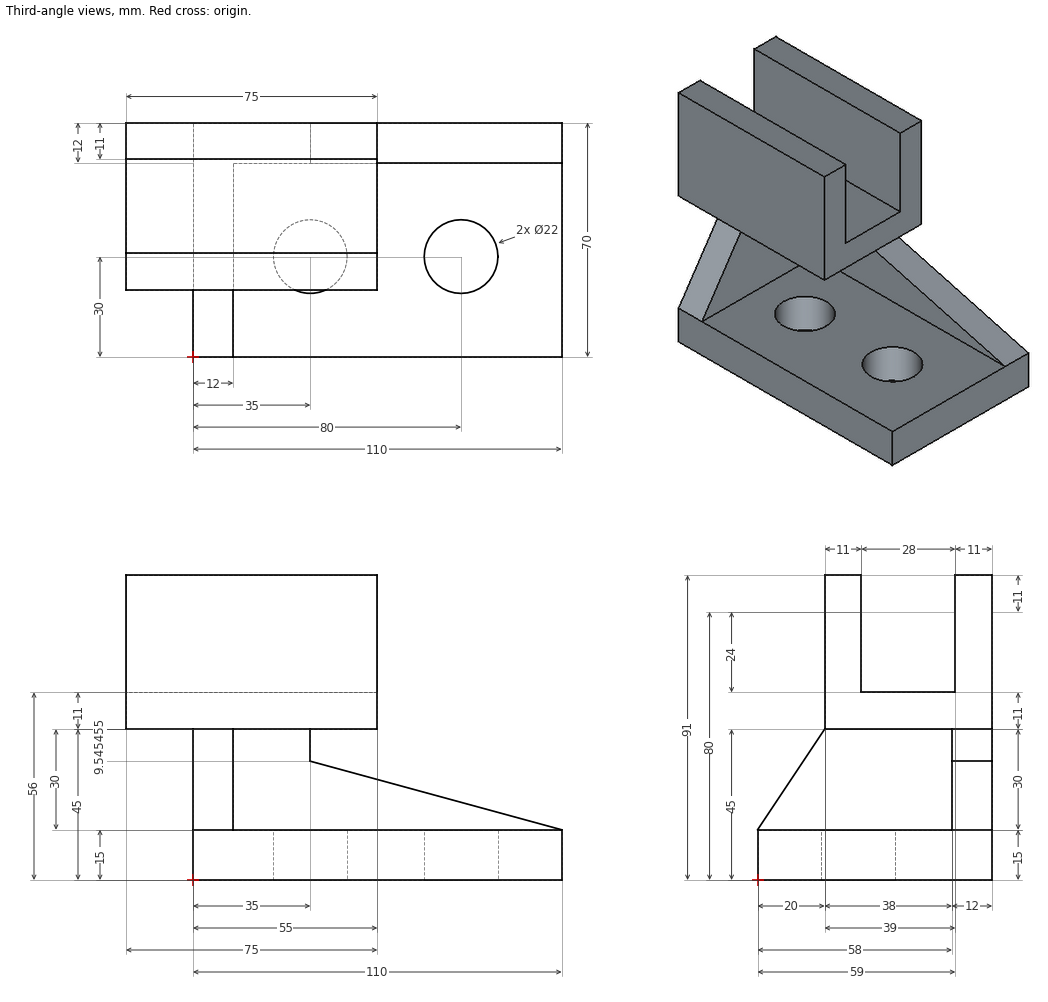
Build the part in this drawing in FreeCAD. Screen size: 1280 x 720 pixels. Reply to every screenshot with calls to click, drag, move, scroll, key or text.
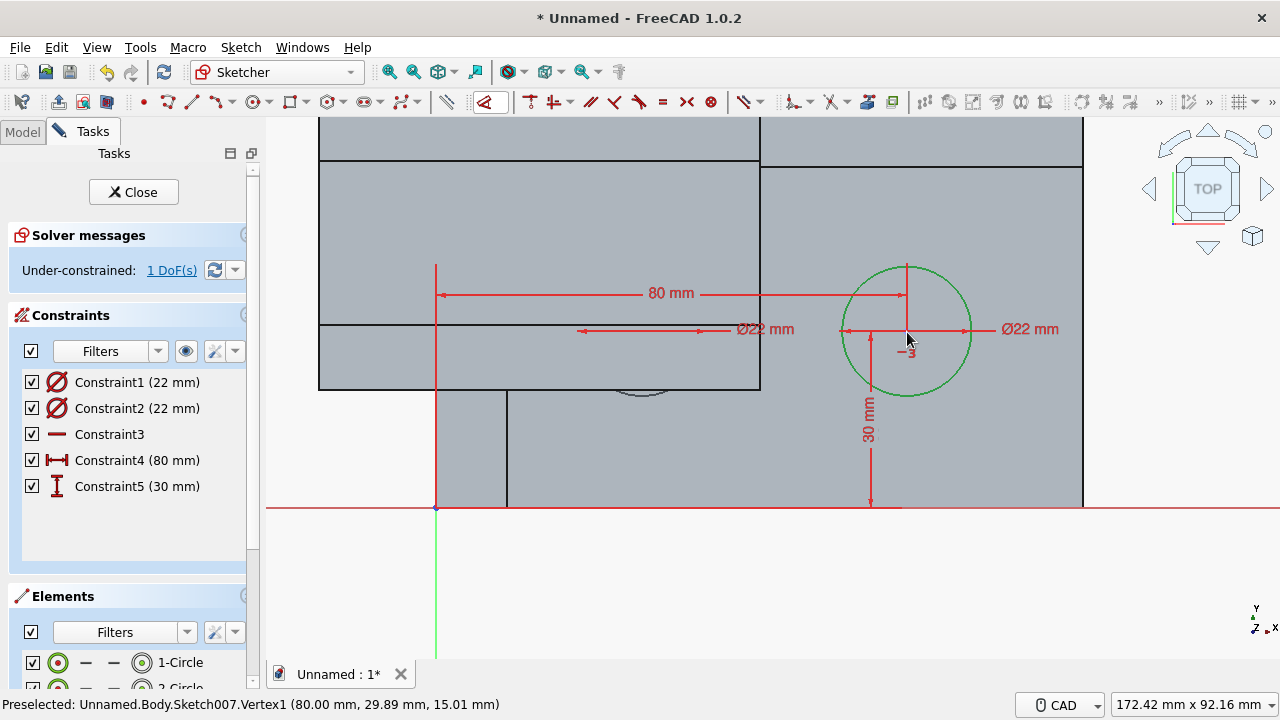
click(642, 331)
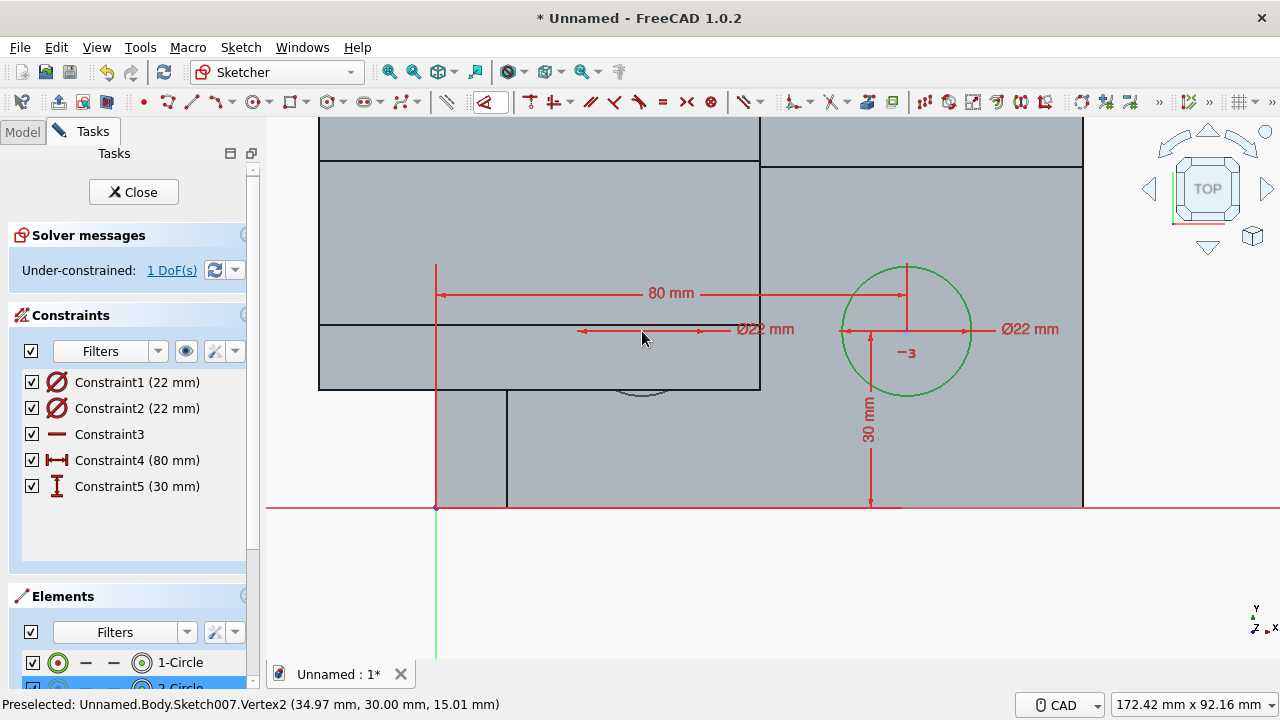
key(l)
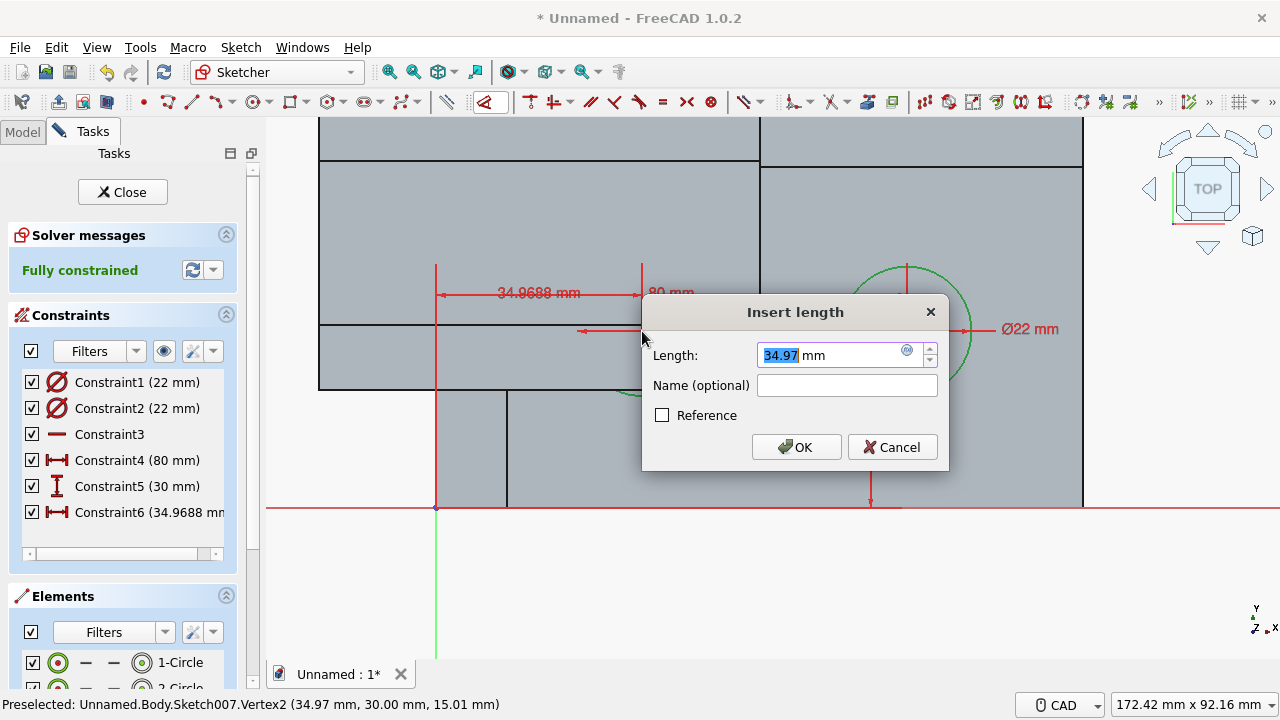
text(35)
key(Return)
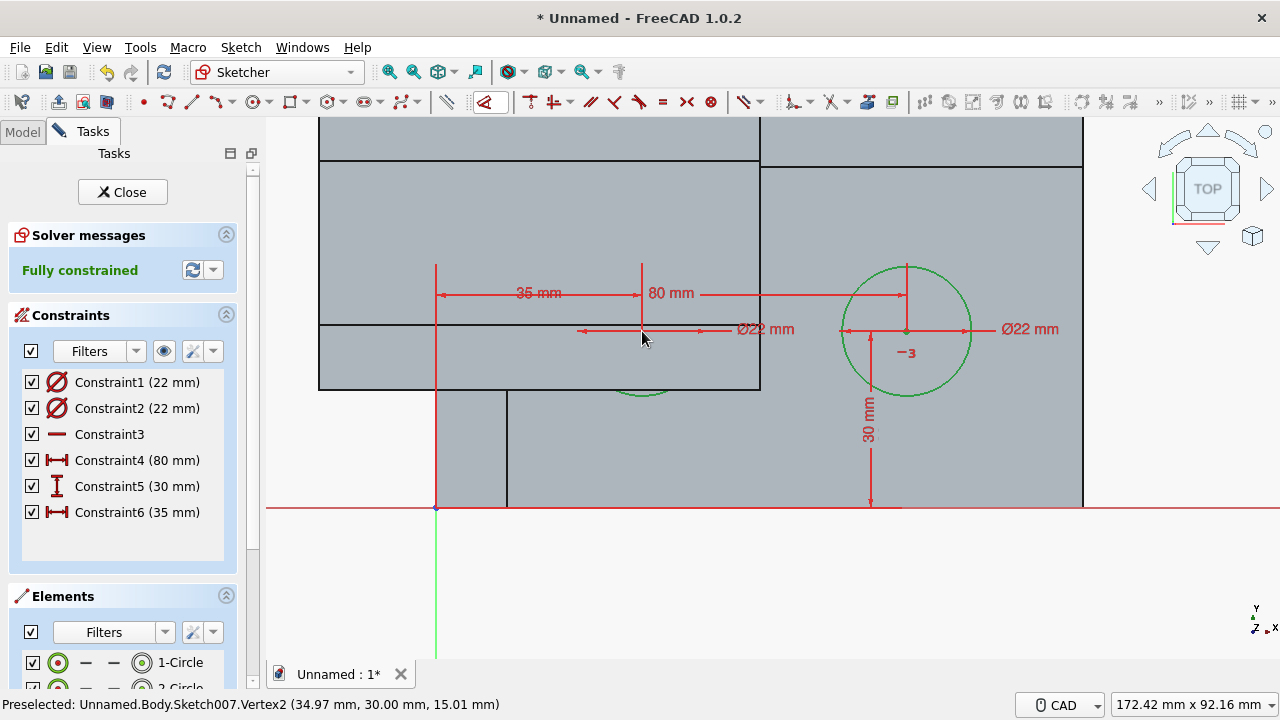
click(123, 192)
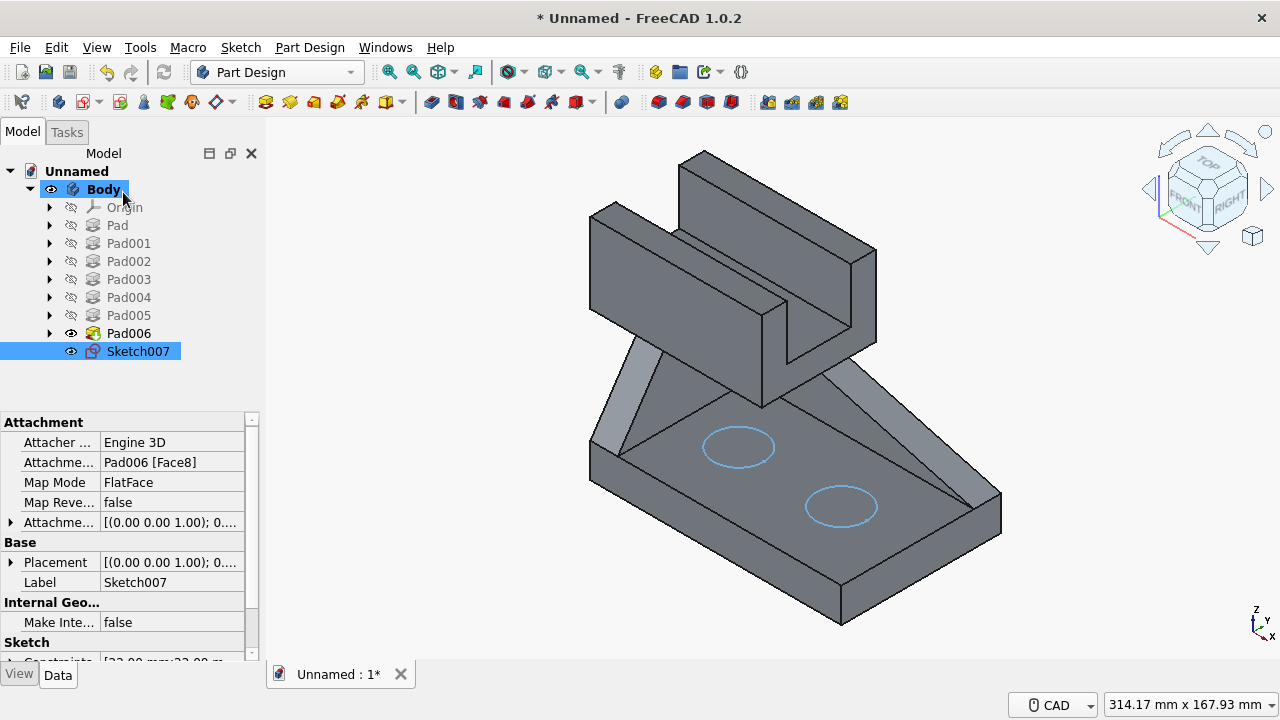
click(432, 102)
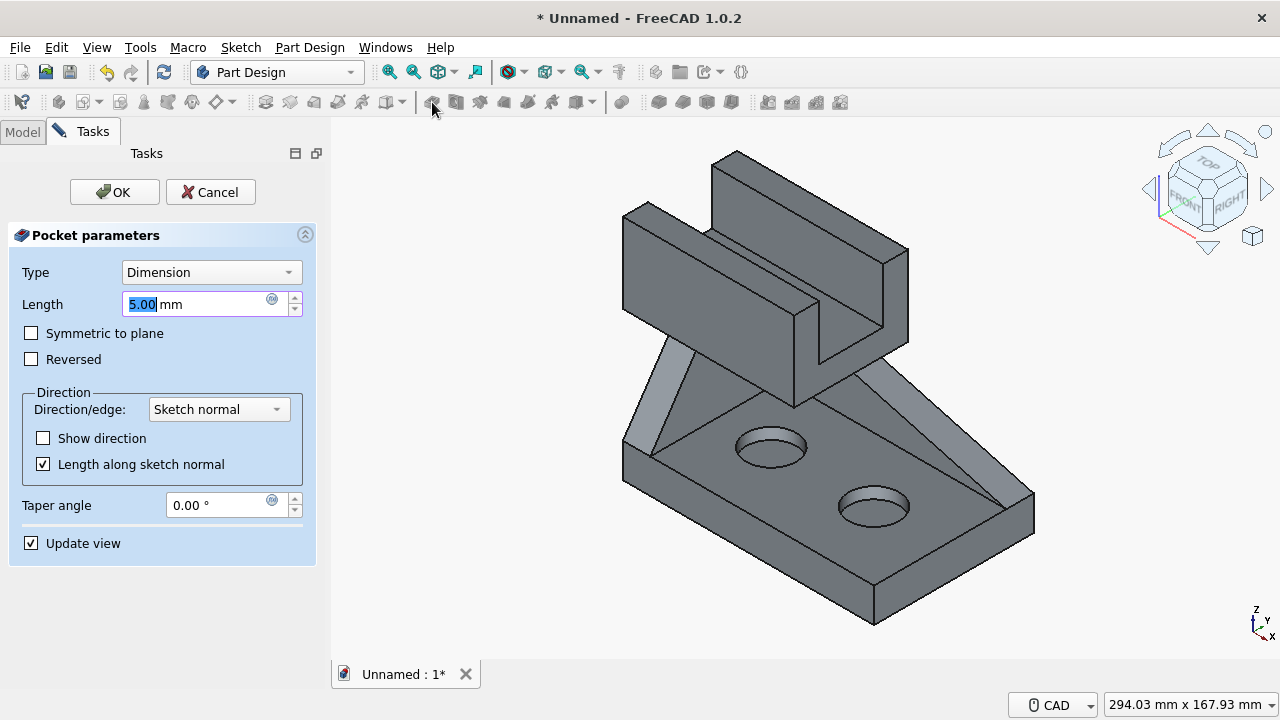
text(15)
key(Tab)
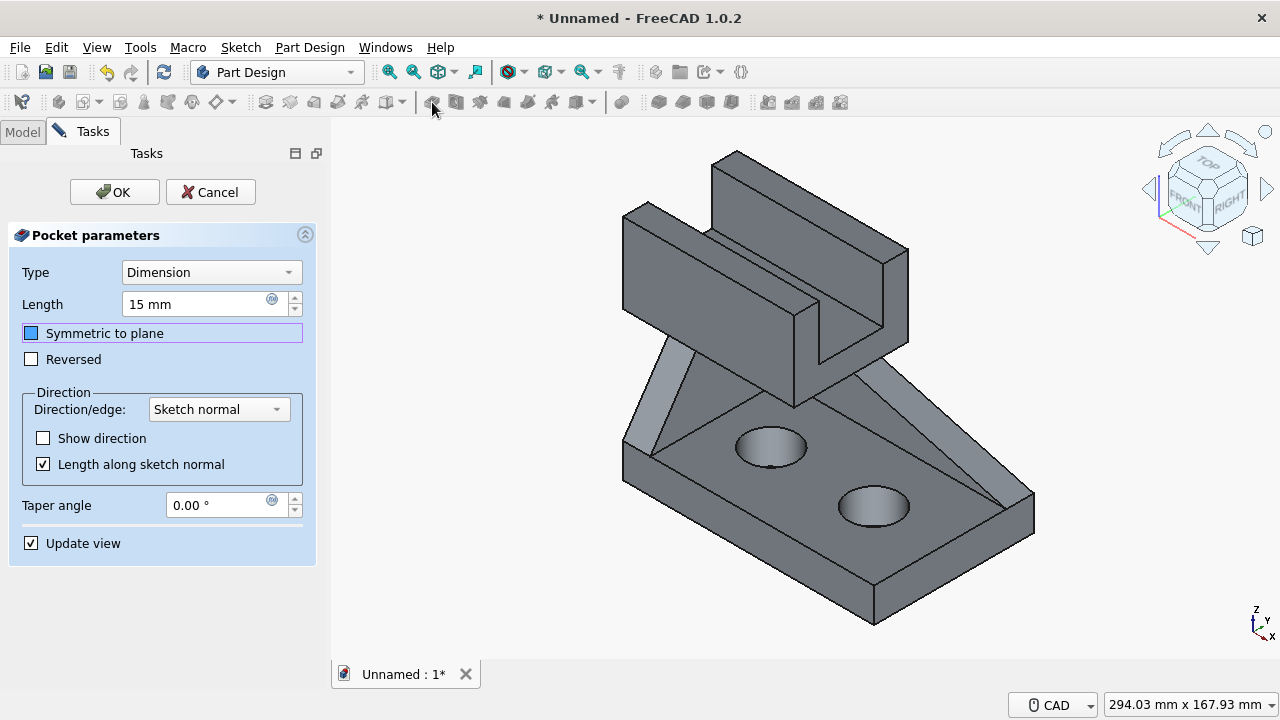
click(115, 192)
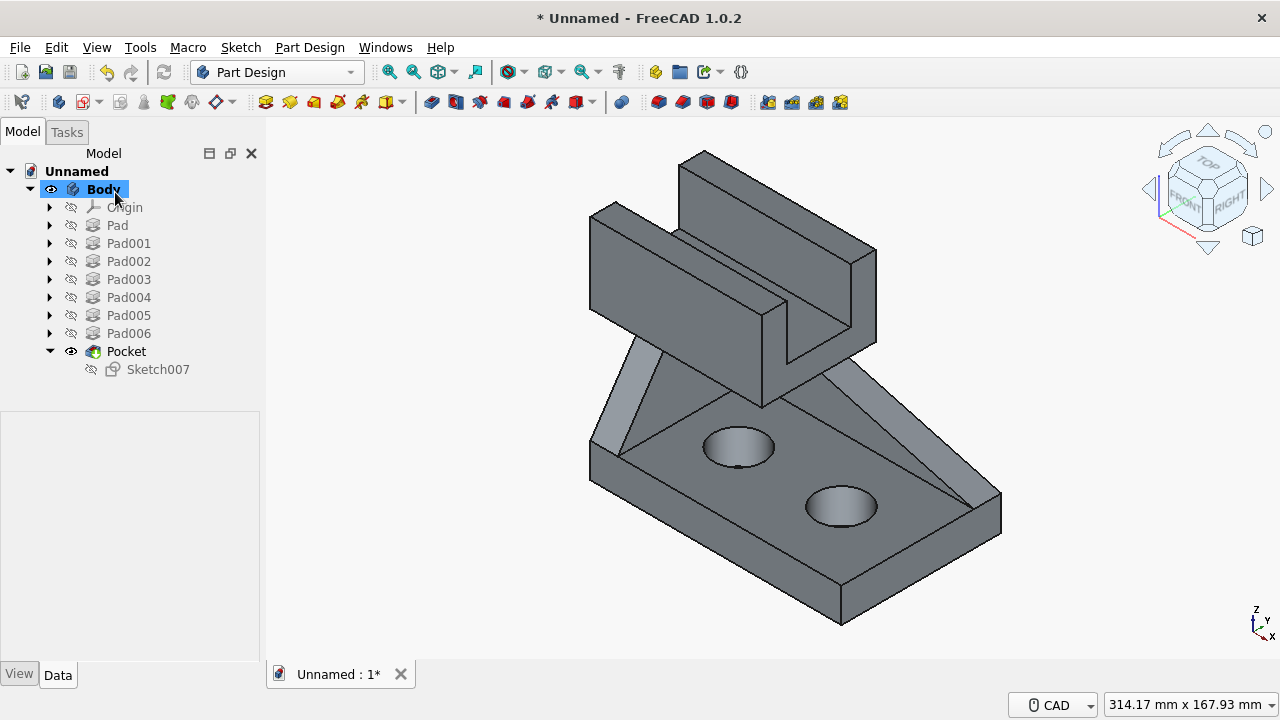
click(770, 330)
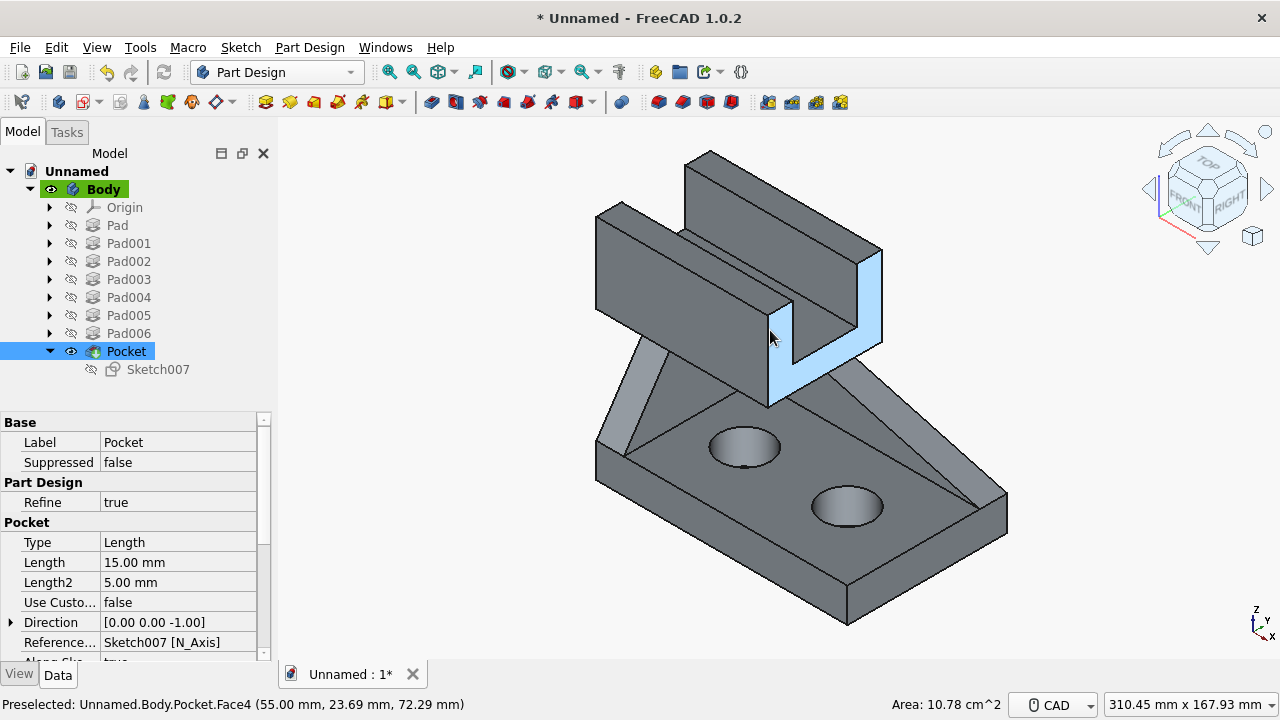
click(84, 102)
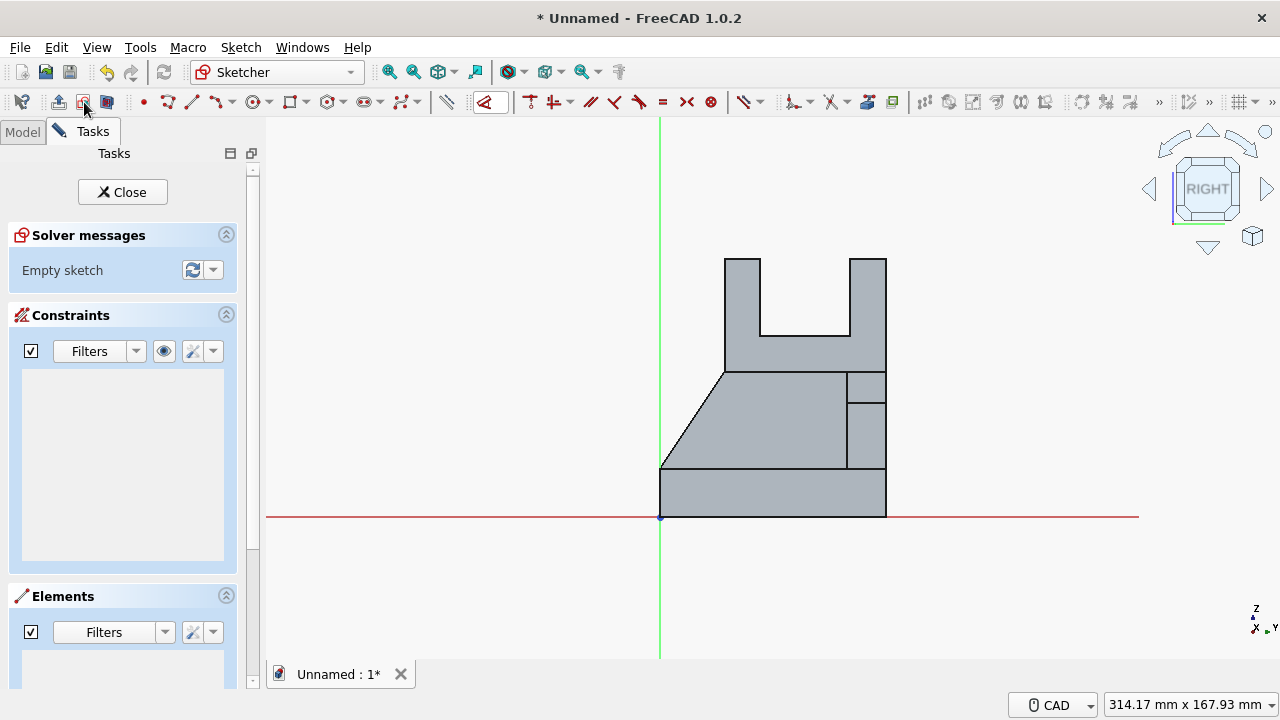
click(108, 102)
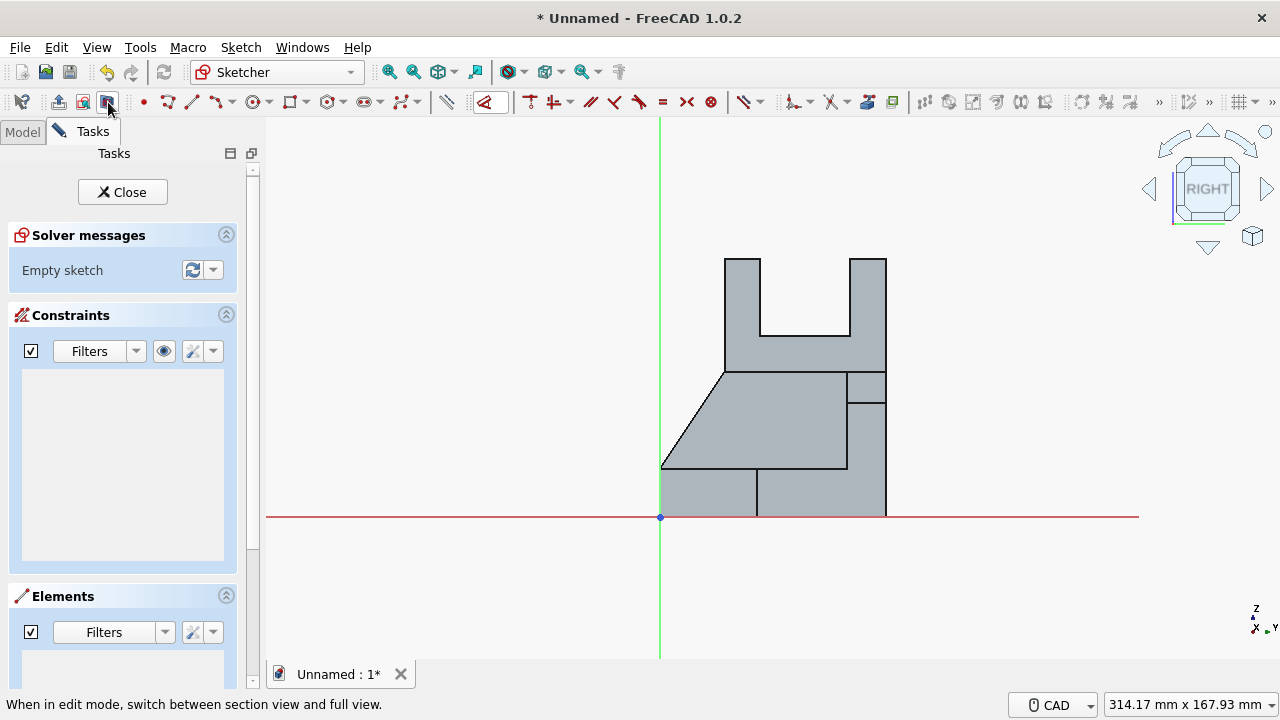
scroll(889, 223, up, 11)